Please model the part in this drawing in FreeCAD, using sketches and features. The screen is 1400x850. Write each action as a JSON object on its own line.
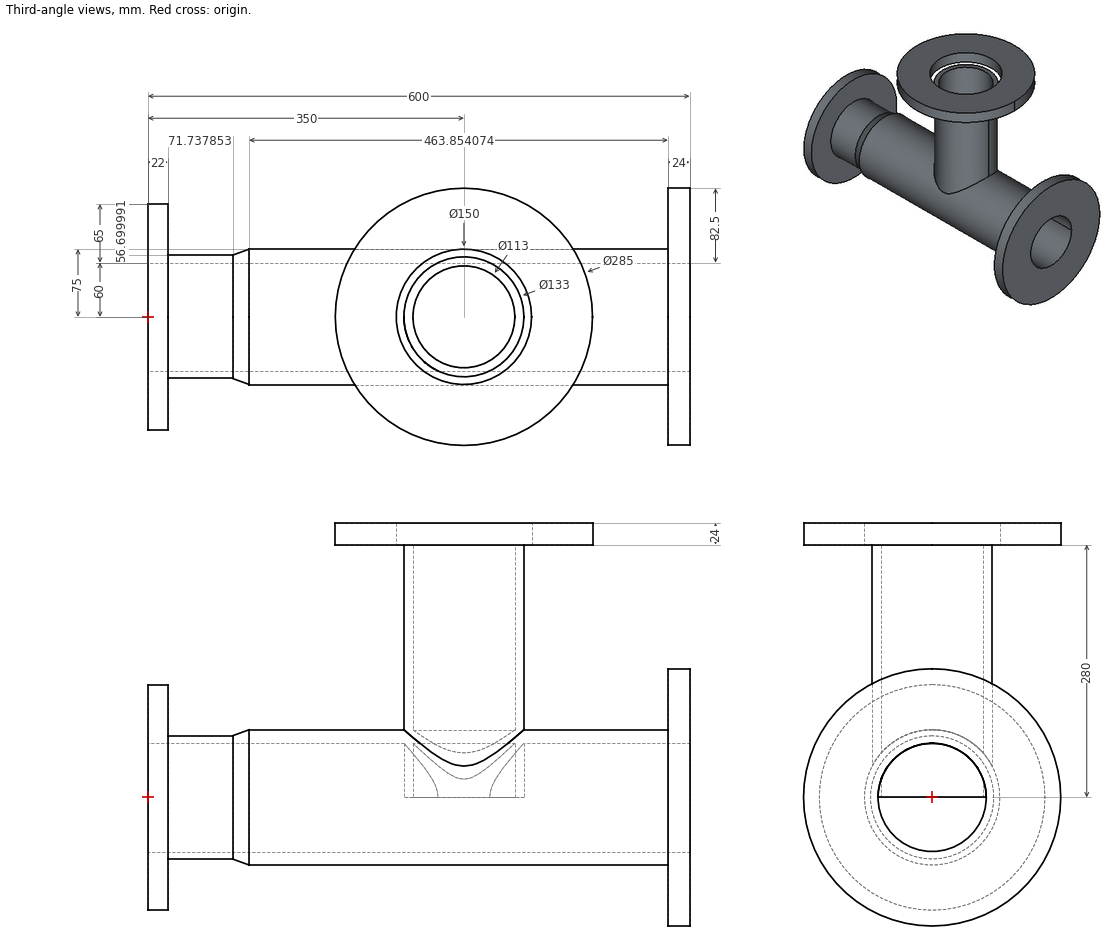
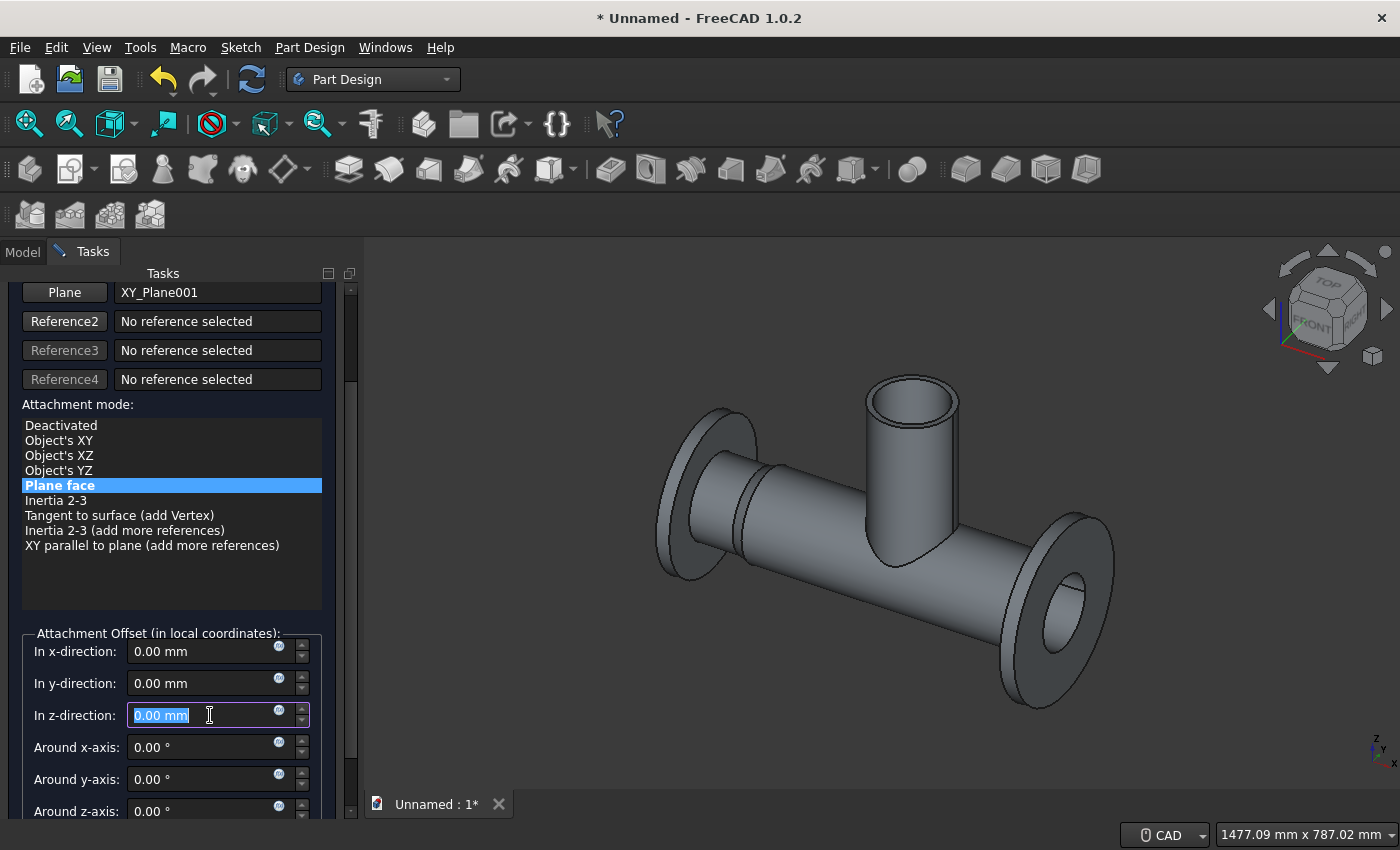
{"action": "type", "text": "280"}
{"action": "key", "text": "Tab"}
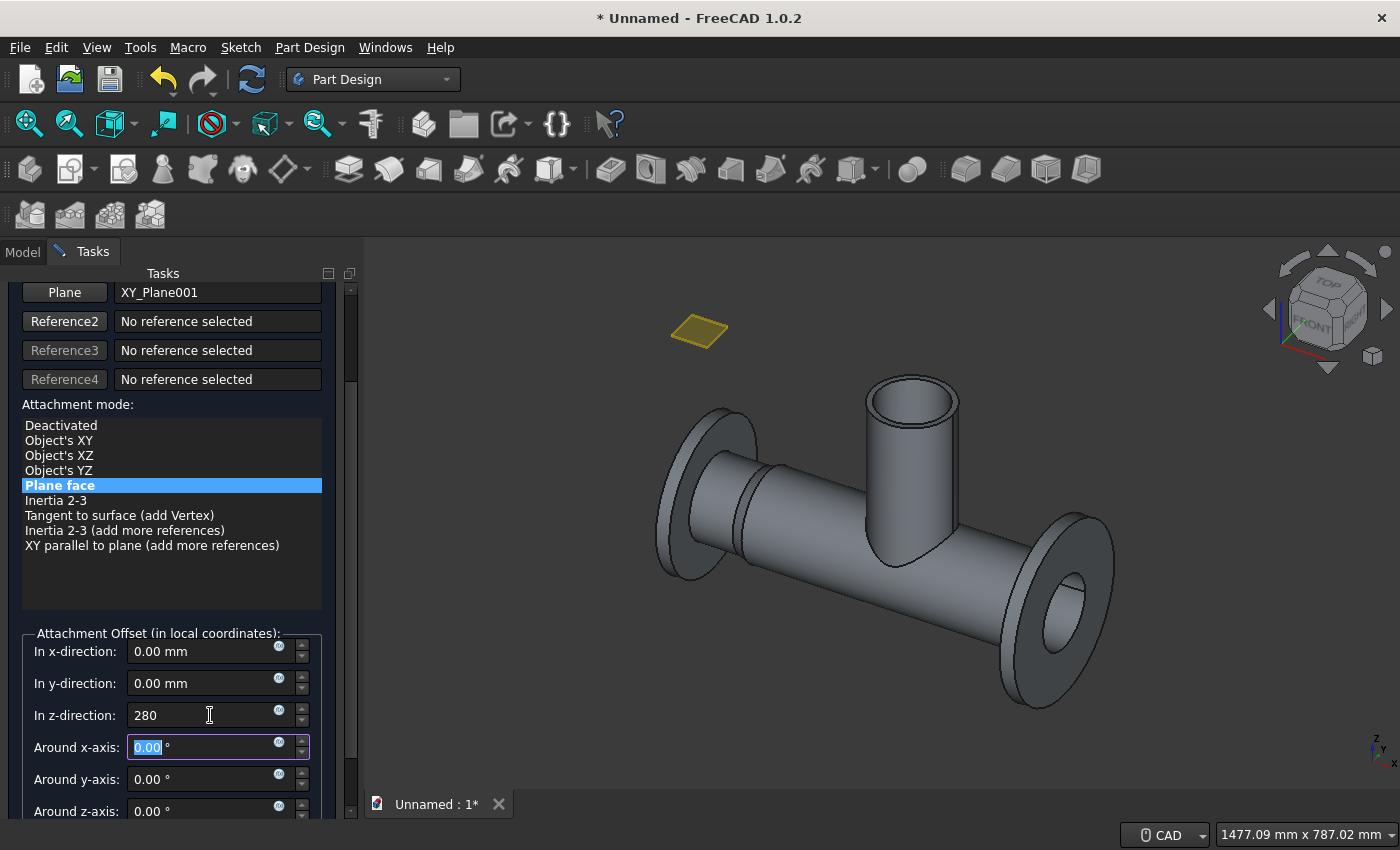
{"action": "scroll", "coordinate": [351, 550], "scroll_direction": "up", "scroll_amount": 3}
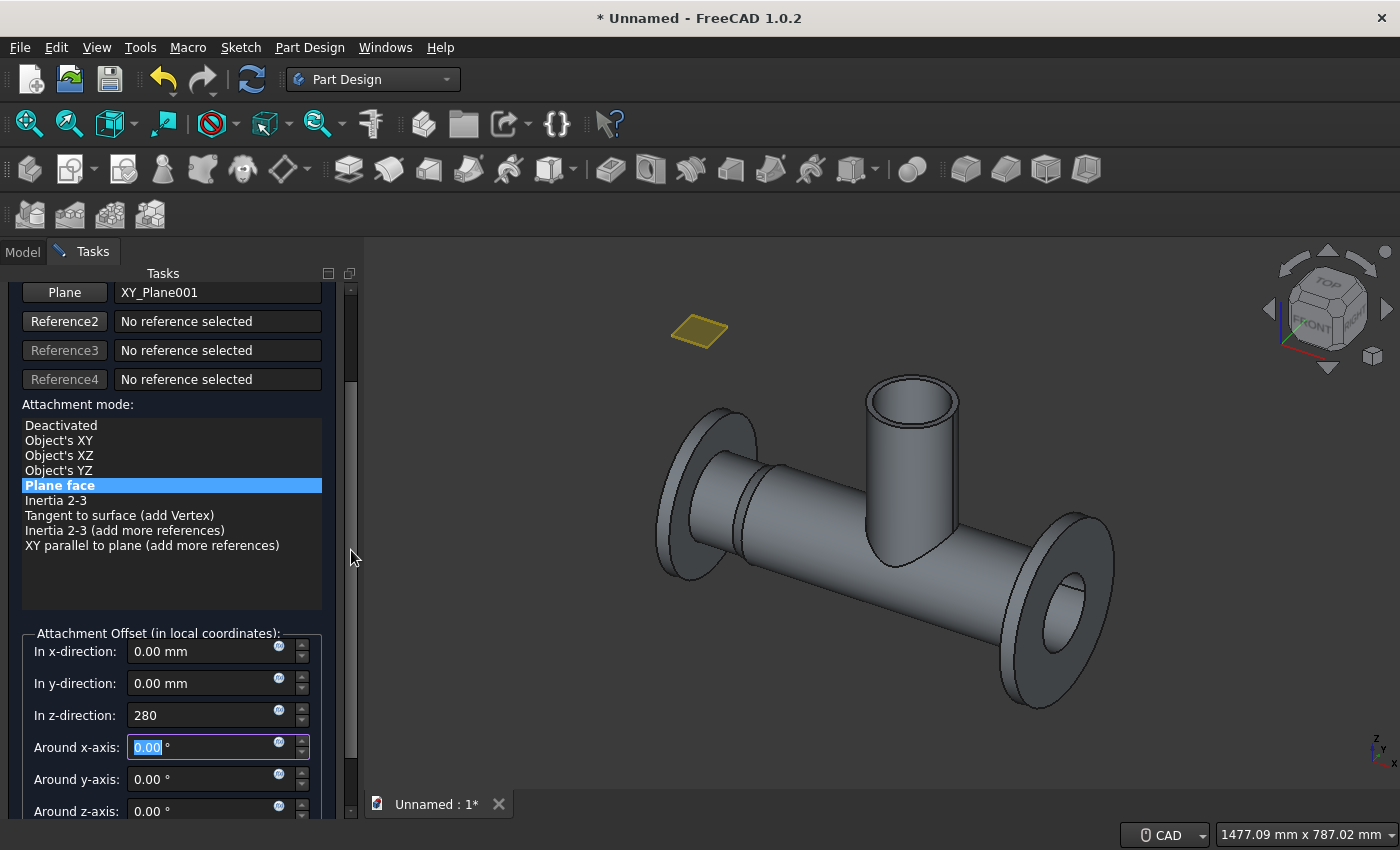
{"action": "left_click", "coordinate": [124, 312]}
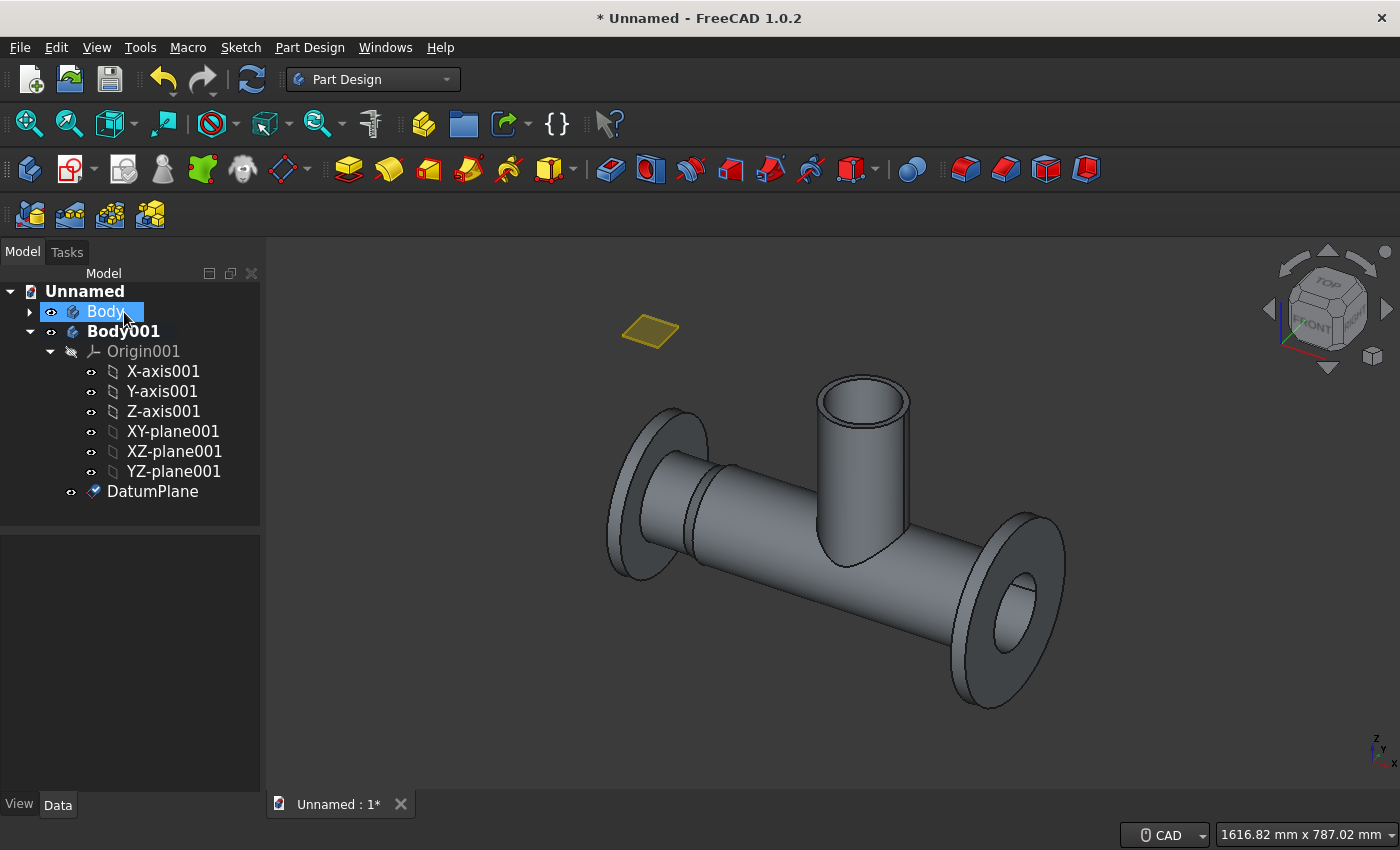
{"action": "left_click", "coordinate": [116, 492]}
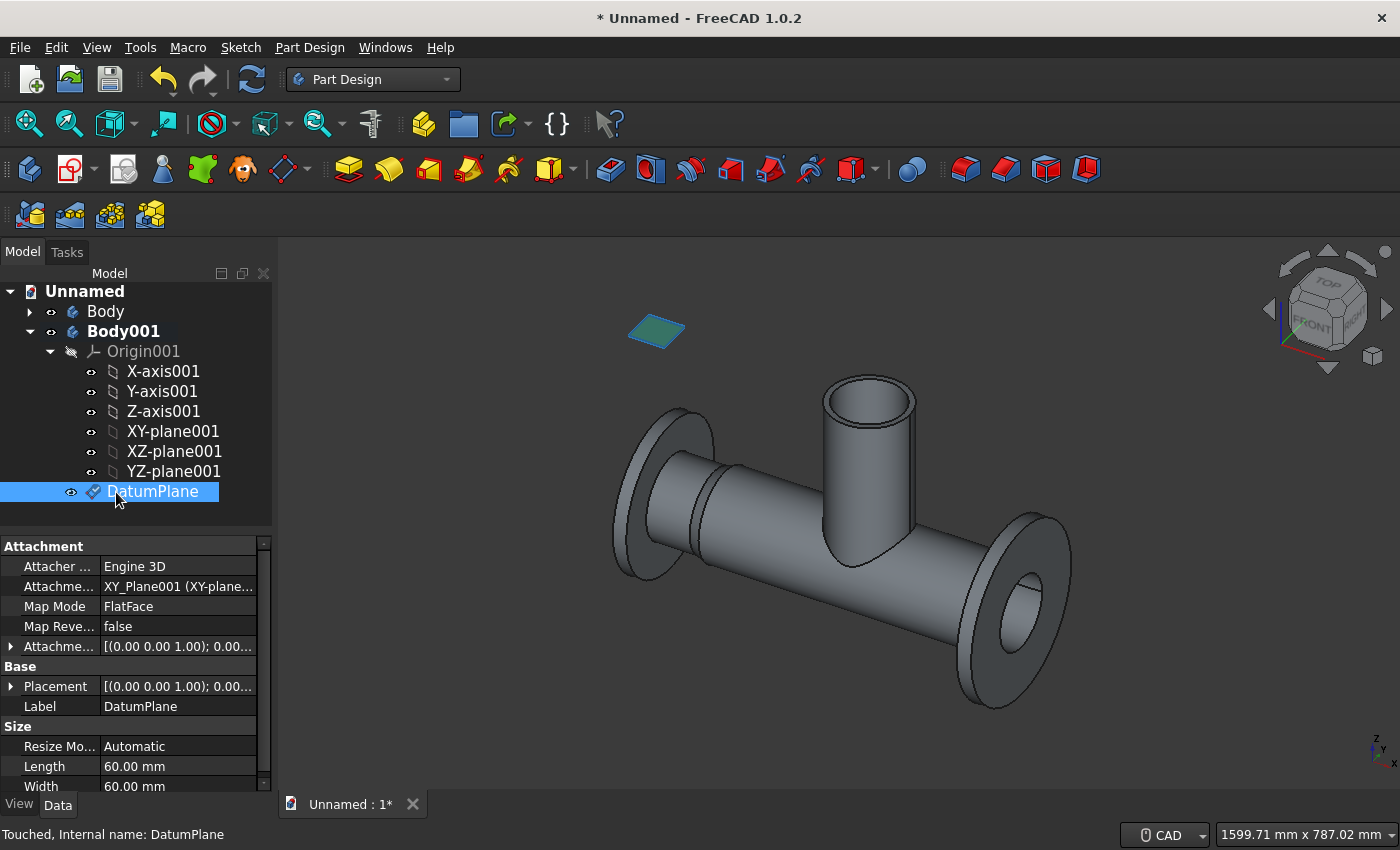
{"action": "left_click", "coordinate": [70, 170]}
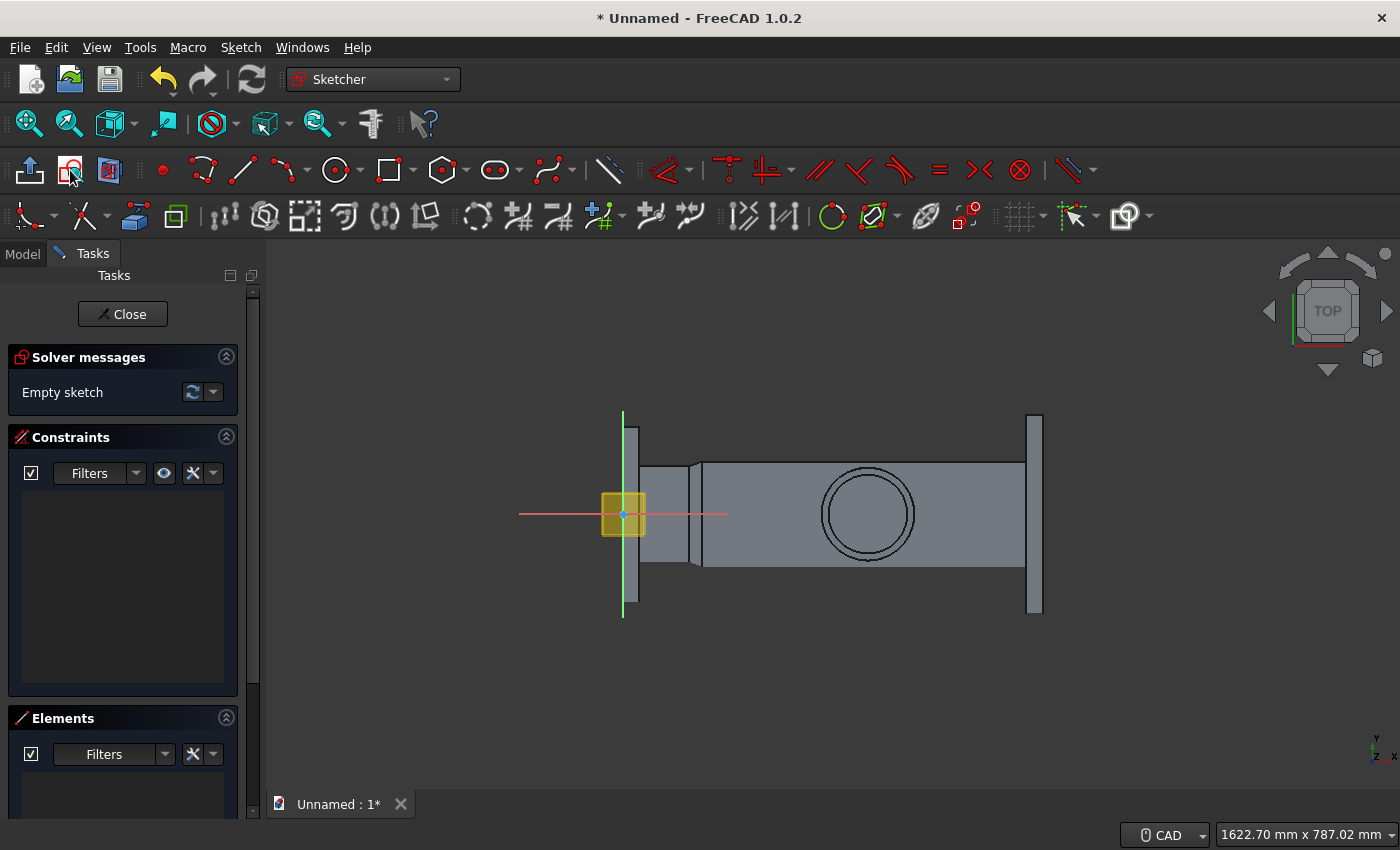
{"action": "scroll", "coordinate": [833, 514], "scroll_direction": "up", "scroll_amount": 3}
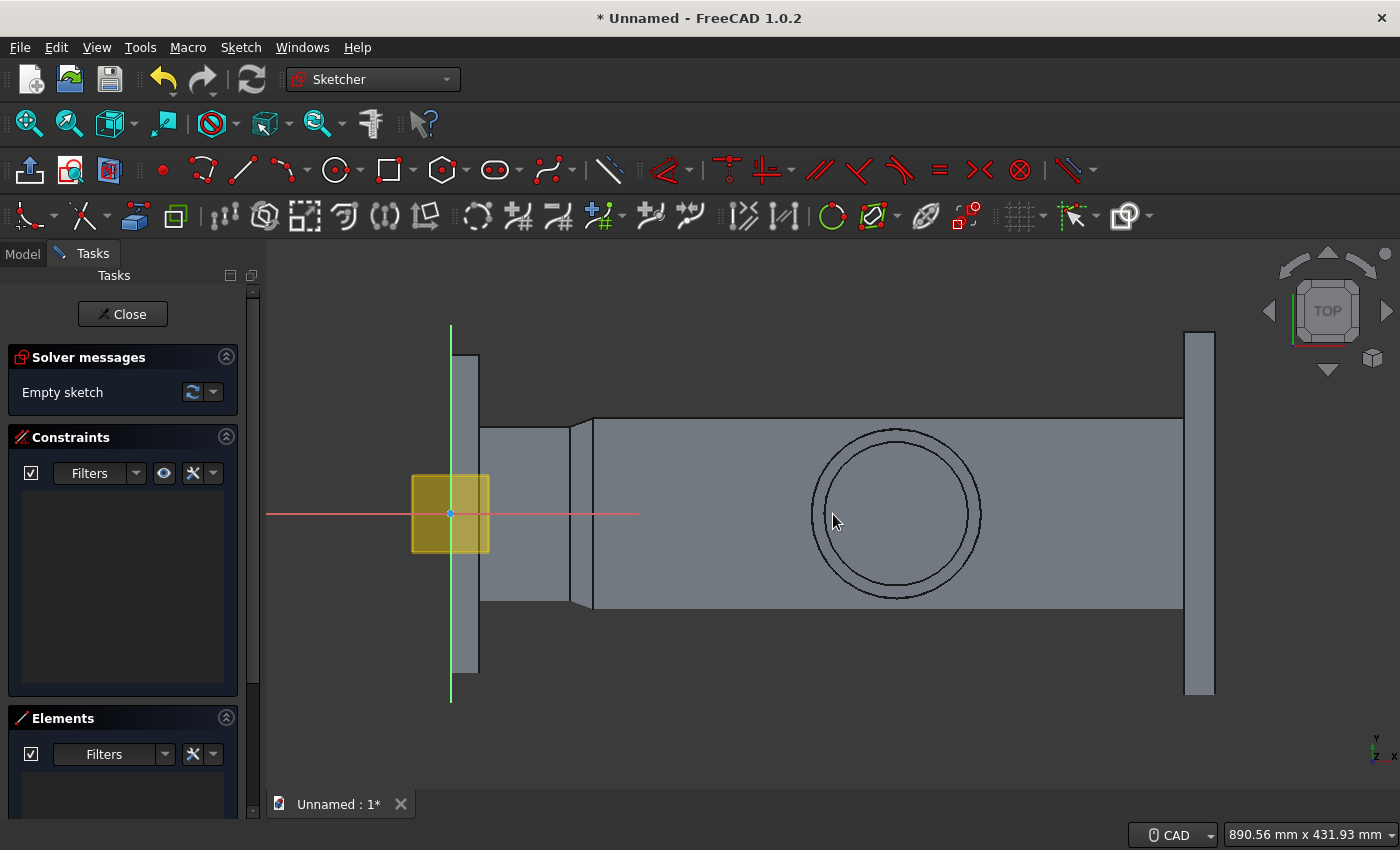
{"action": "key", "text": "g c"}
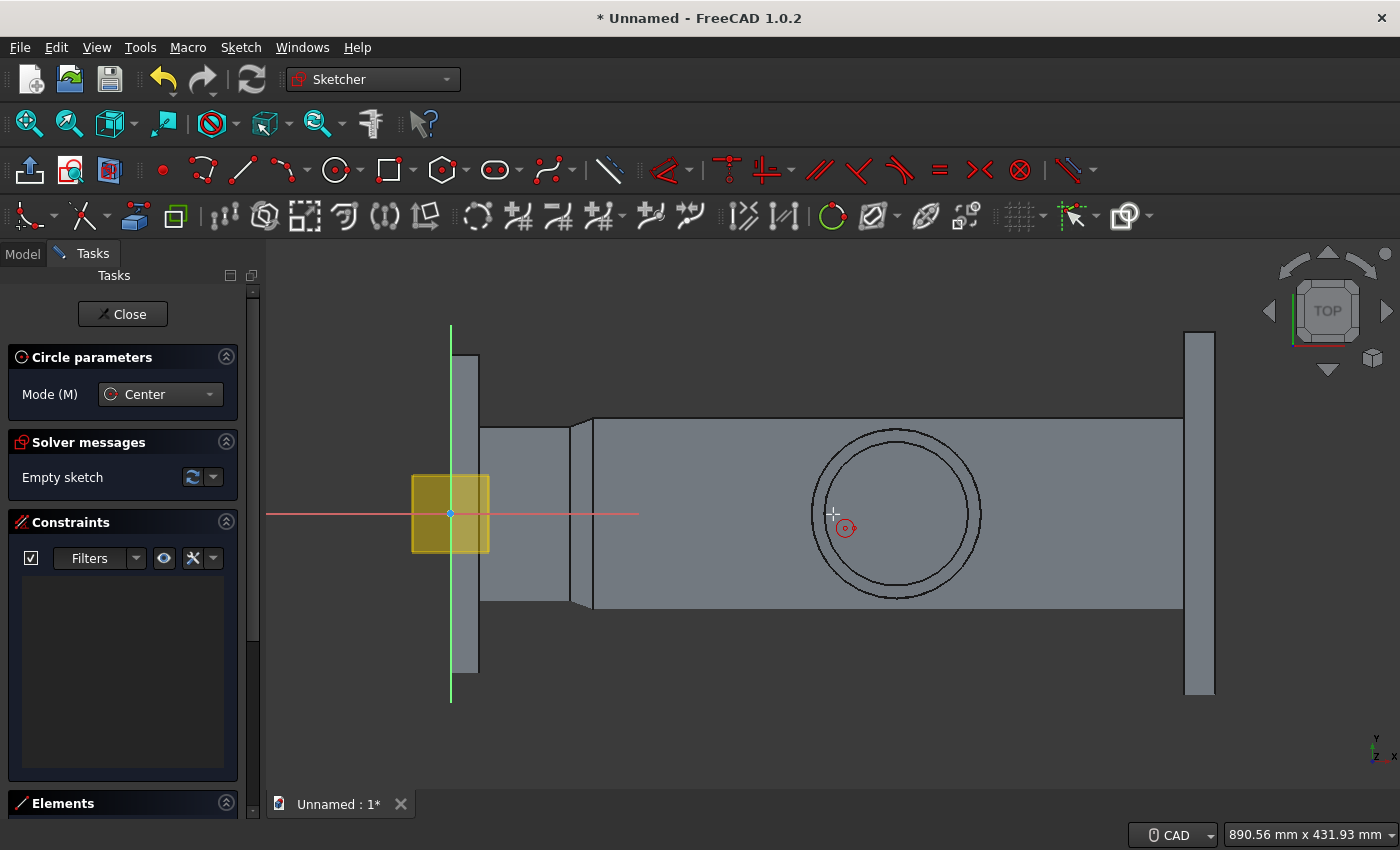
{"action": "left_click", "coordinate": [896, 514]}
{"action": "mouse_move", "coordinate": [1025, 386]}